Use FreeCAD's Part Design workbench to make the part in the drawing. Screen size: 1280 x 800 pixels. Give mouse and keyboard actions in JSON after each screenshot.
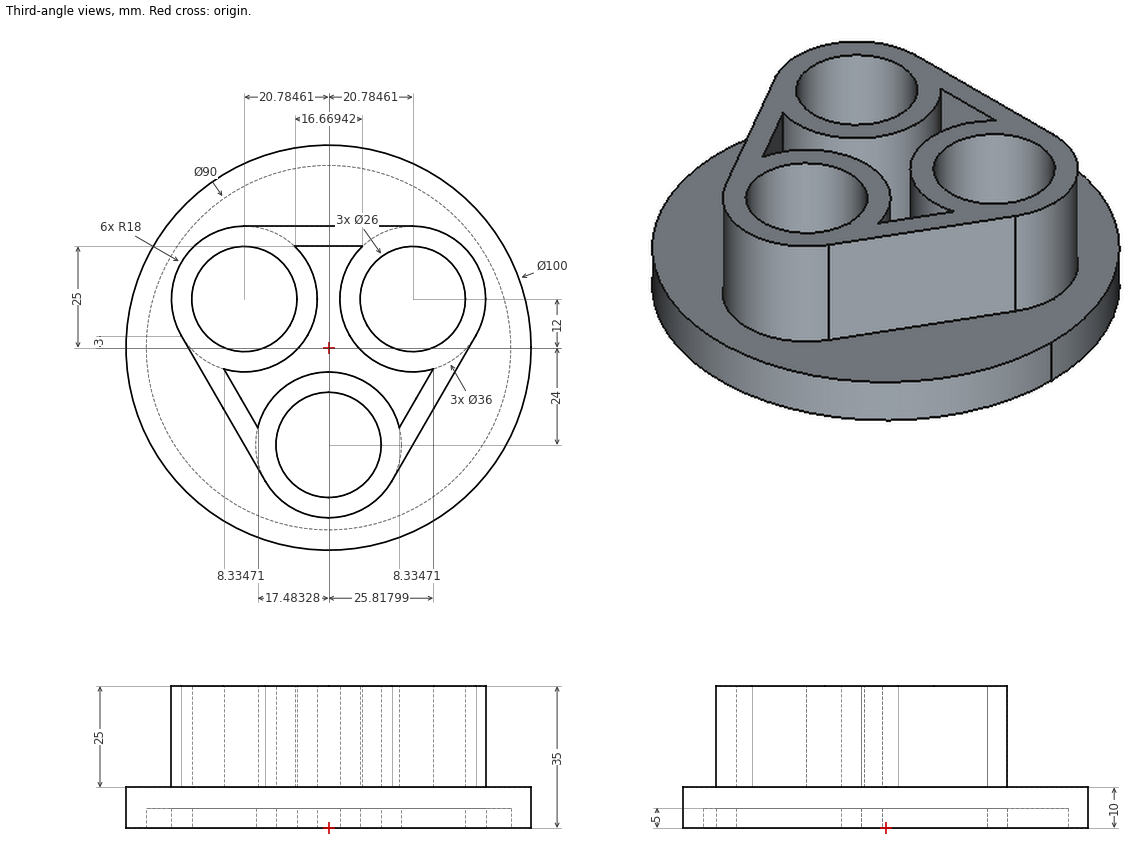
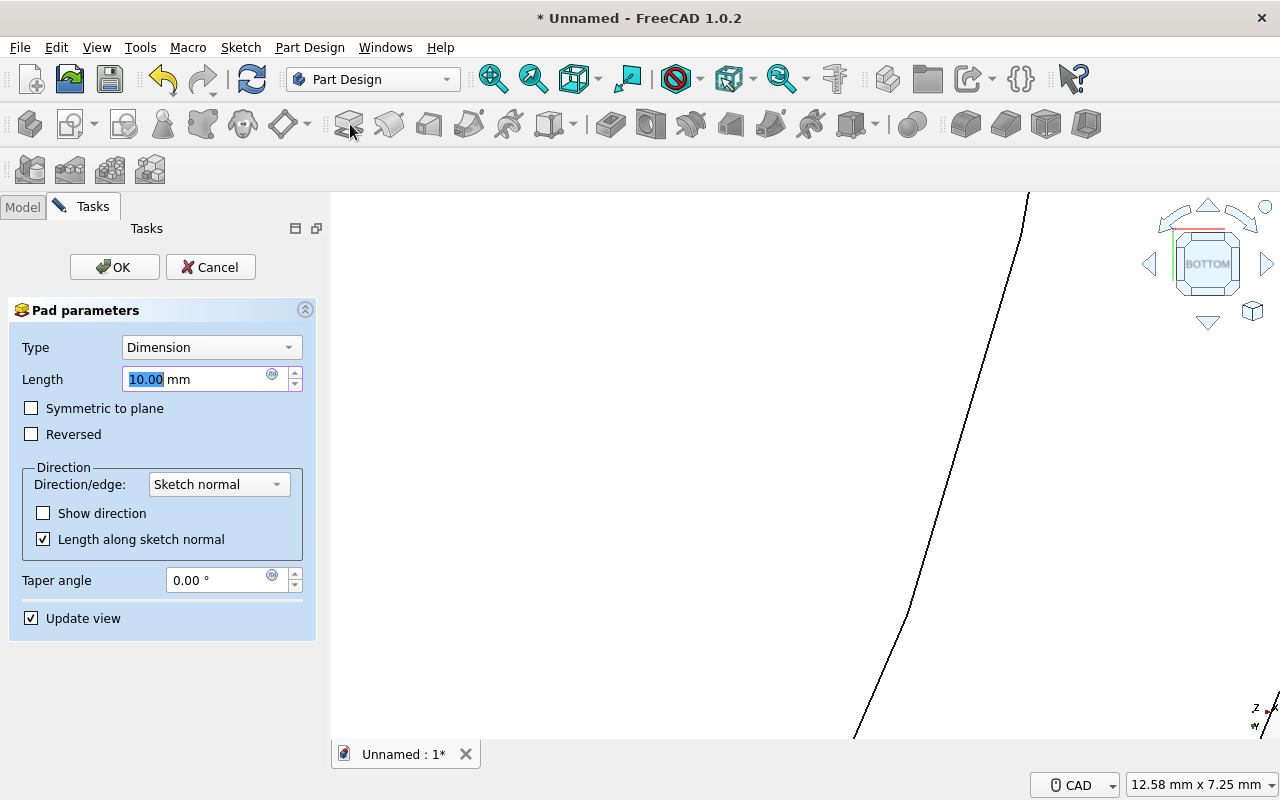
{"action": "type", "text": "35"}
{"action": "key", "text": "Tab"}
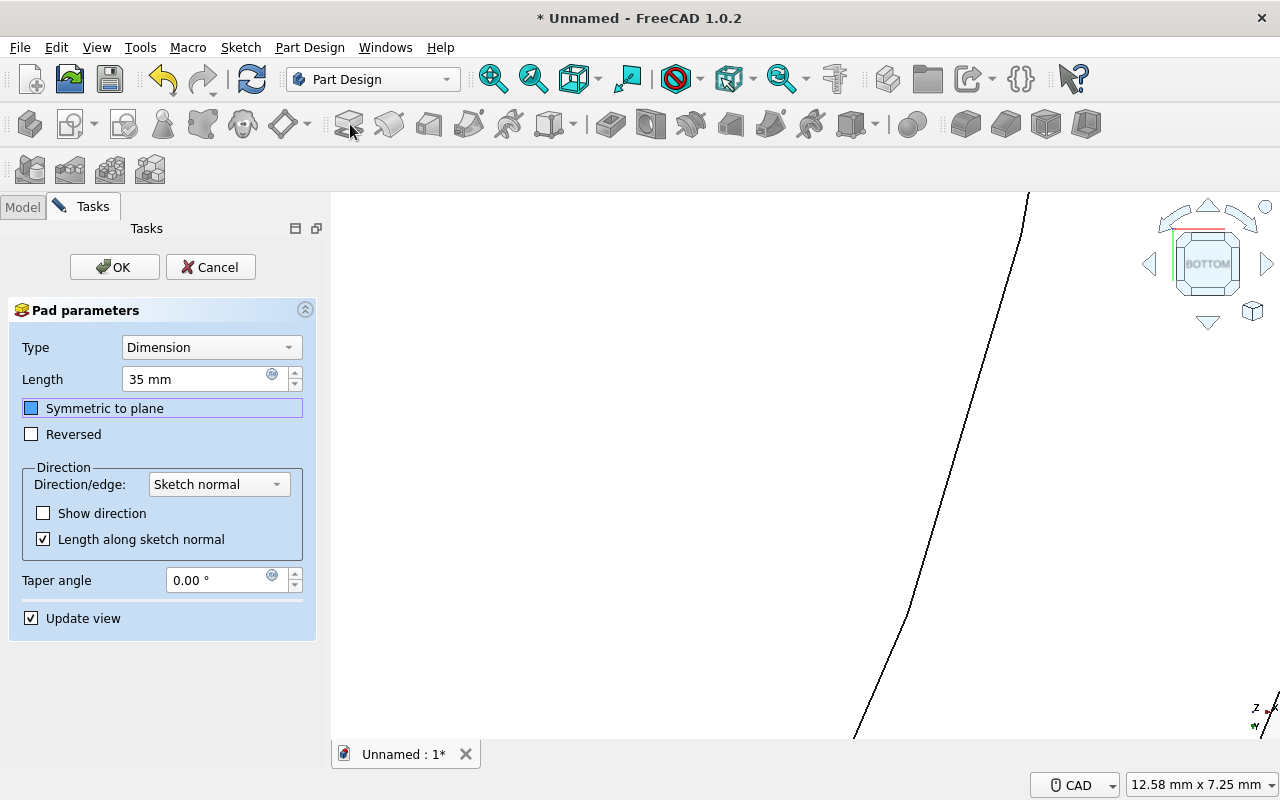
{"action": "left_click", "coordinate": [30, 434]}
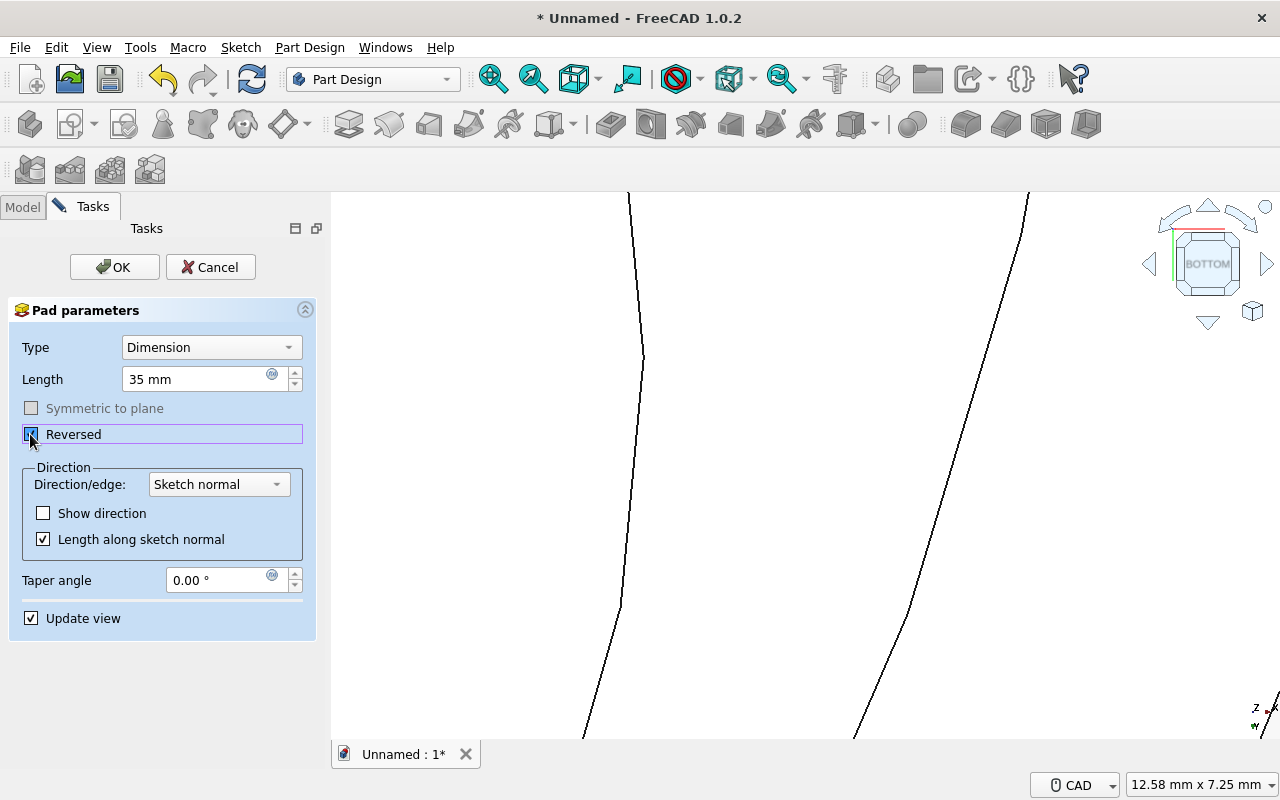
{"action": "left_click", "coordinate": [115, 267]}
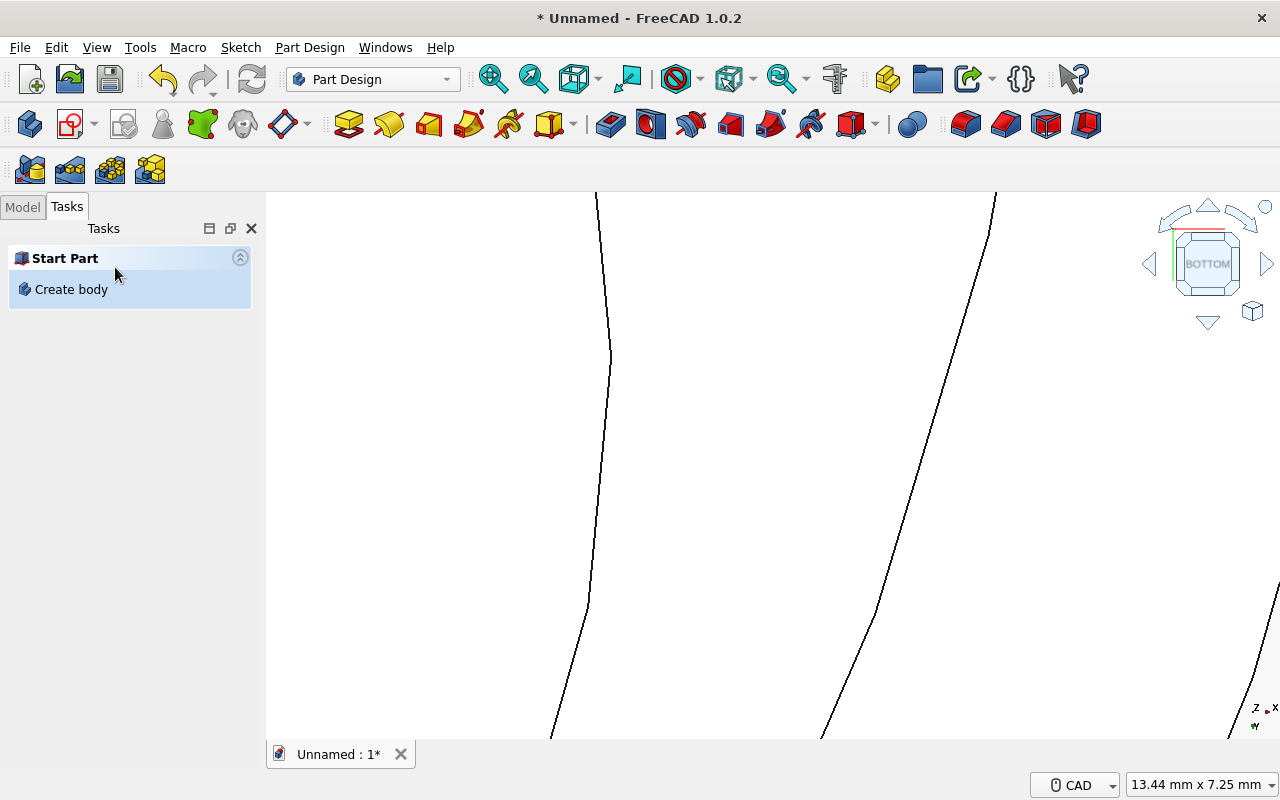
{"action": "key", "text": "0"}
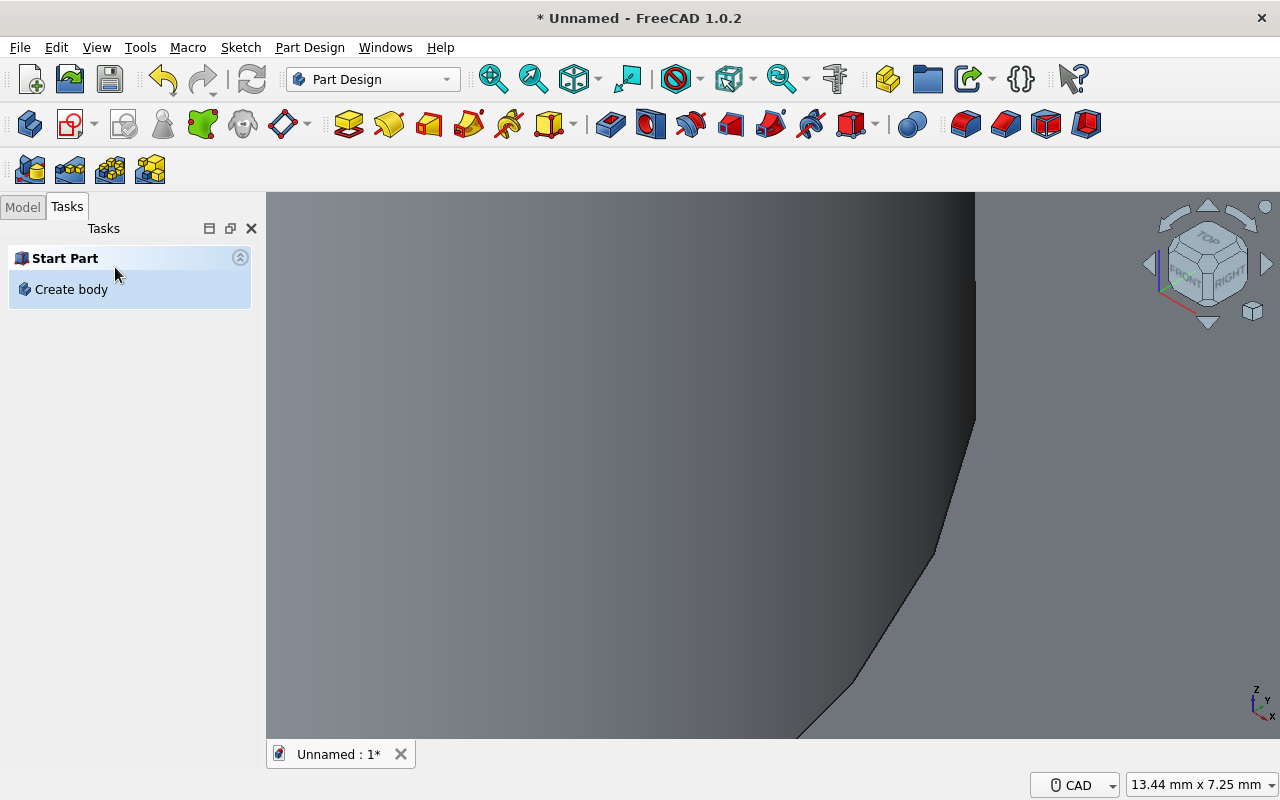
{"action": "left_click", "coordinate": [494, 80]}